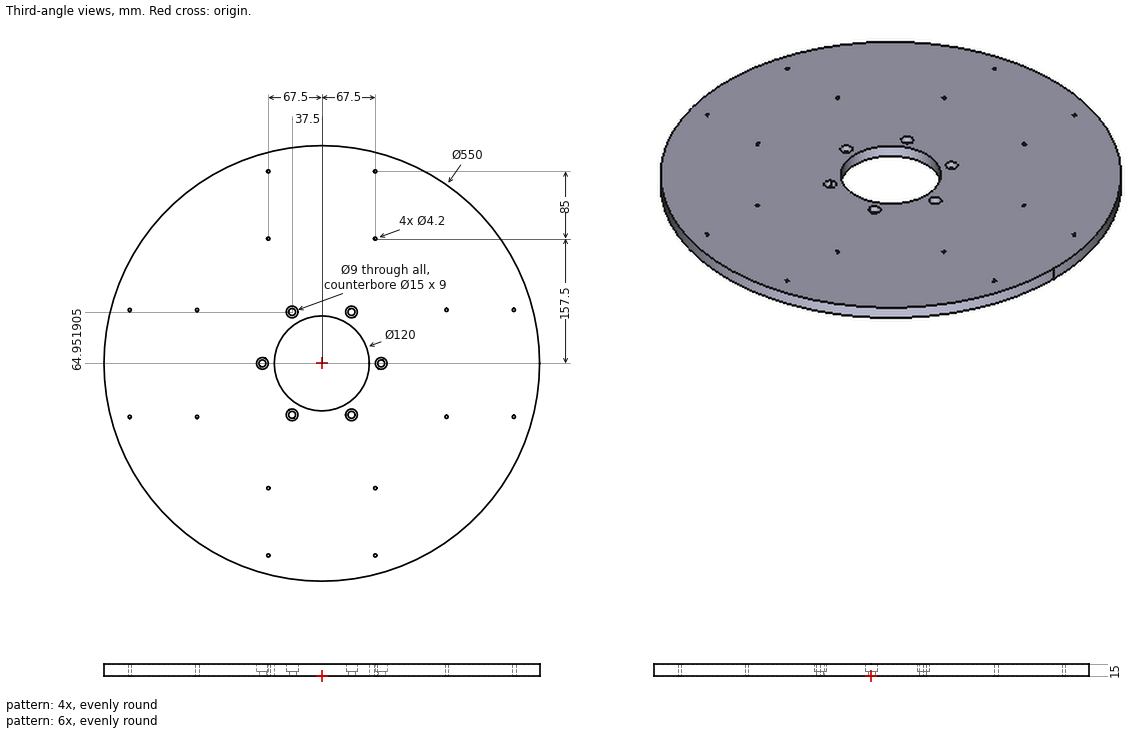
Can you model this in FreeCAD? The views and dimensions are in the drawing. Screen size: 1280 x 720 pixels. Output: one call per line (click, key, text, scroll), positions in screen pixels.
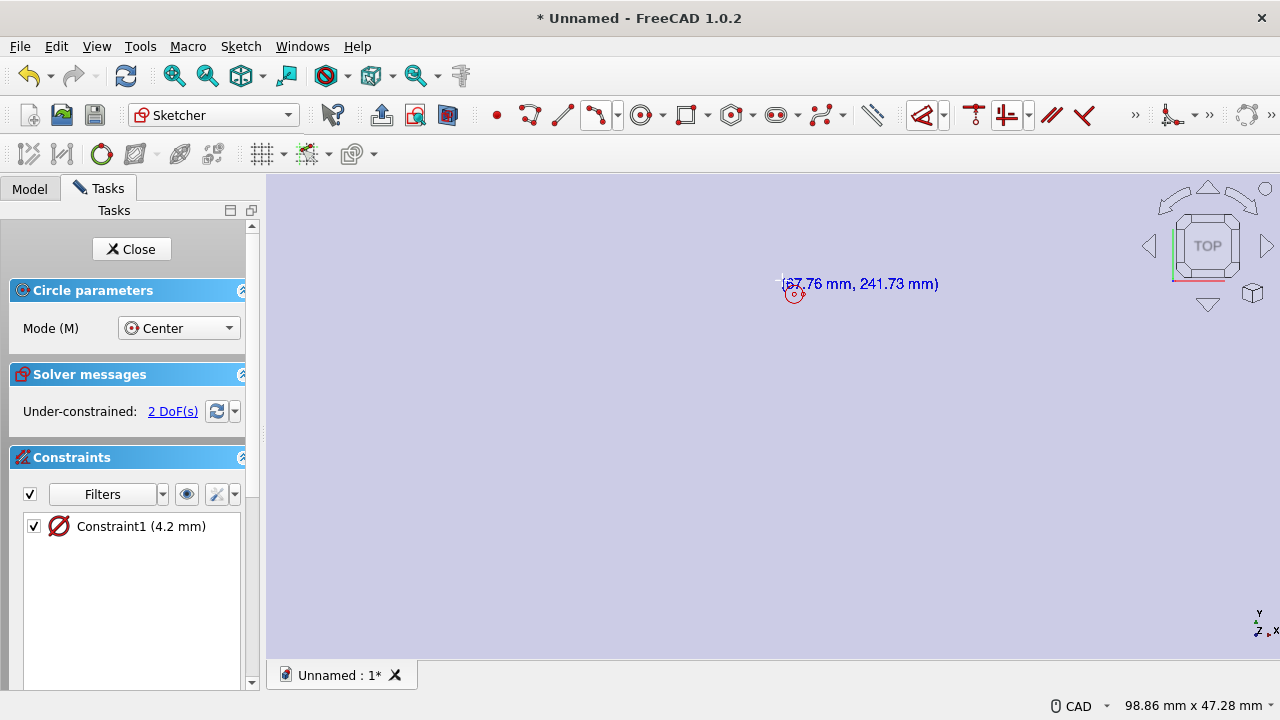
scroll(782, 280, down, 12)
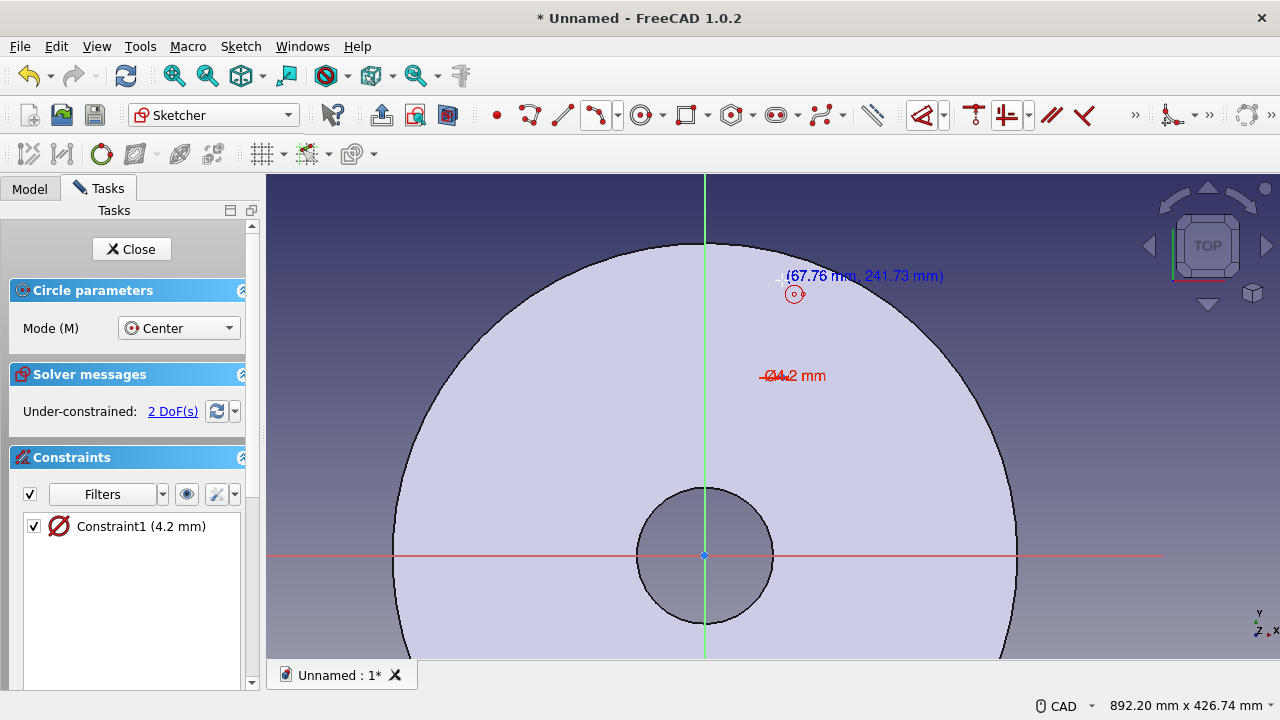
click(782, 280)
move(783, 278)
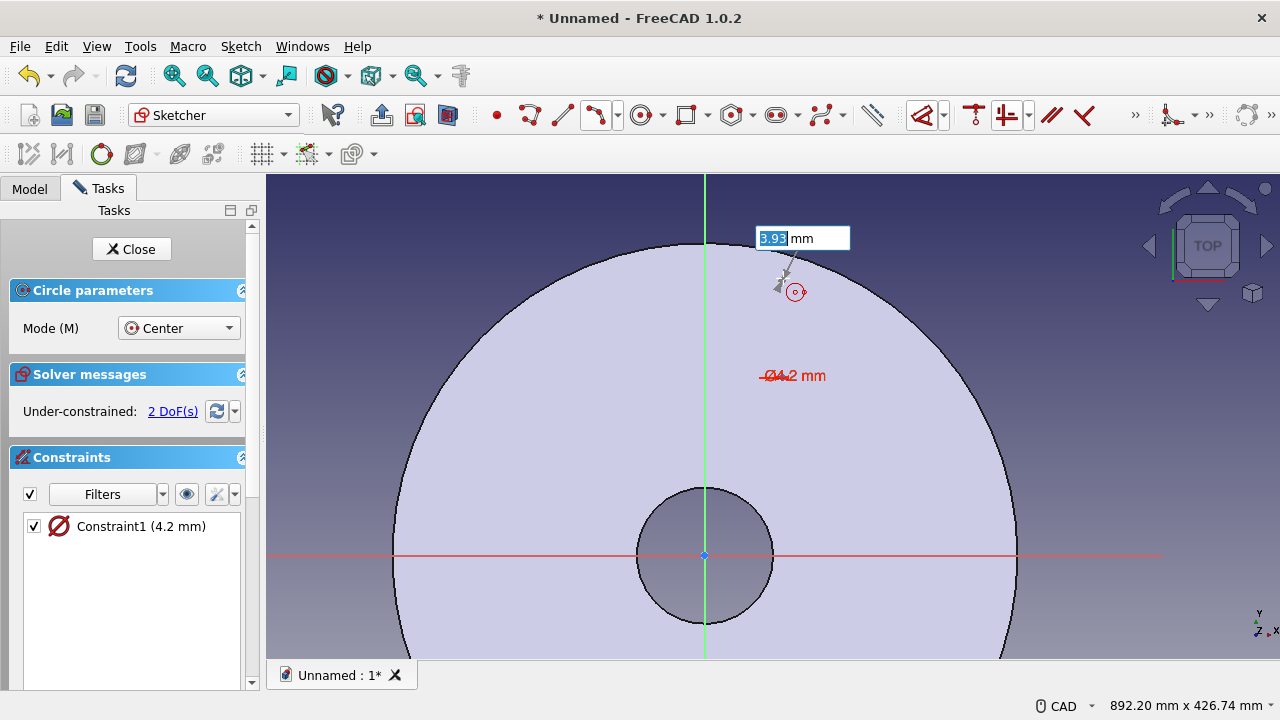
text(4.2)
key(Return)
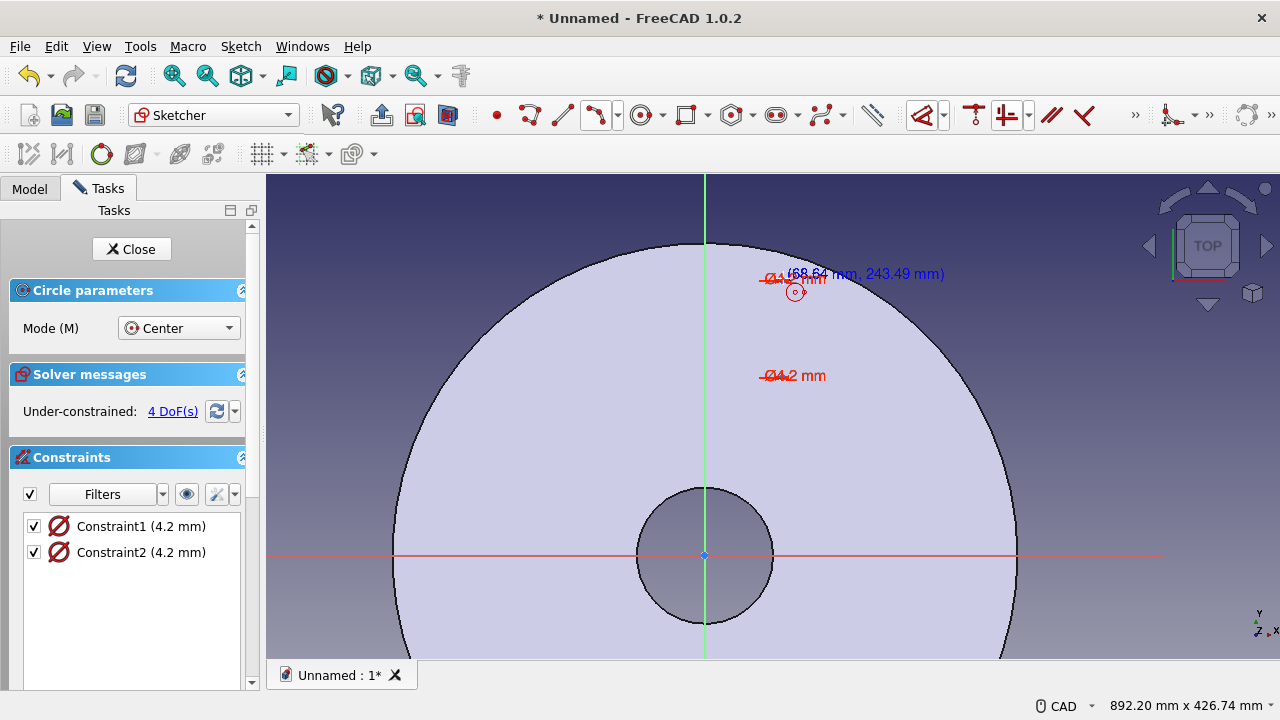
scroll(628, 377, up, 12)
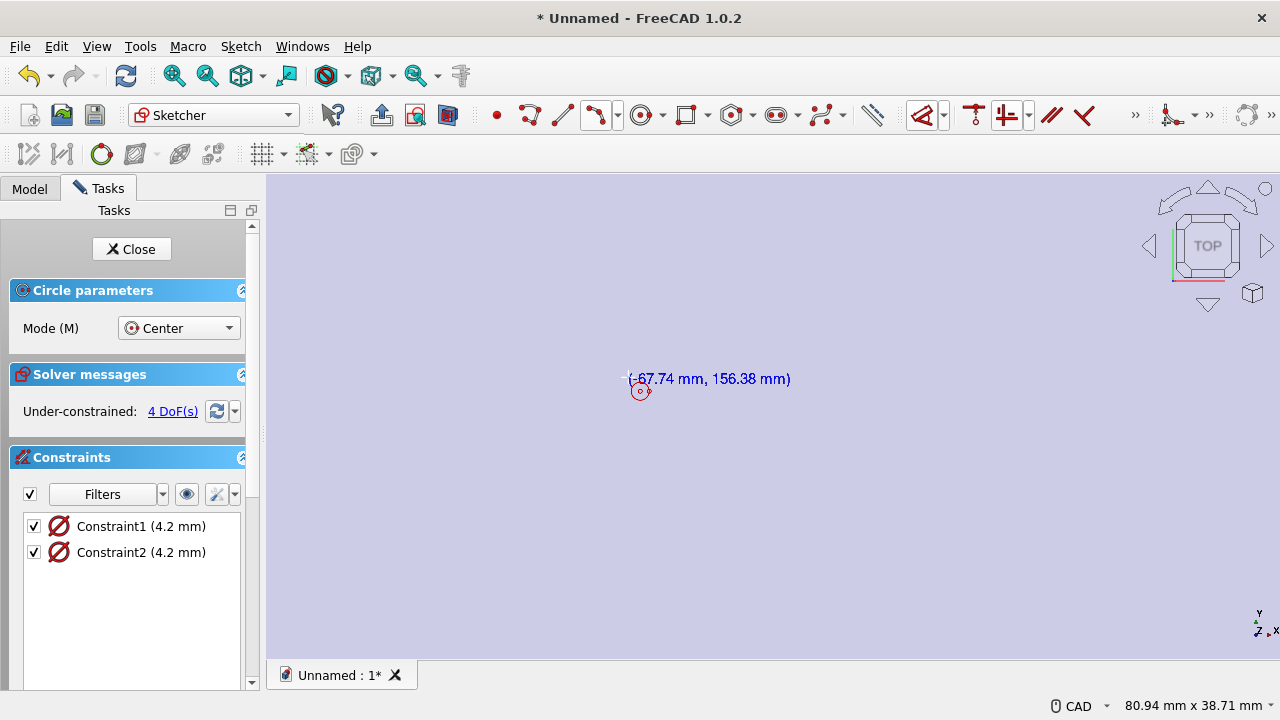
scroll(628, 377, down, 12)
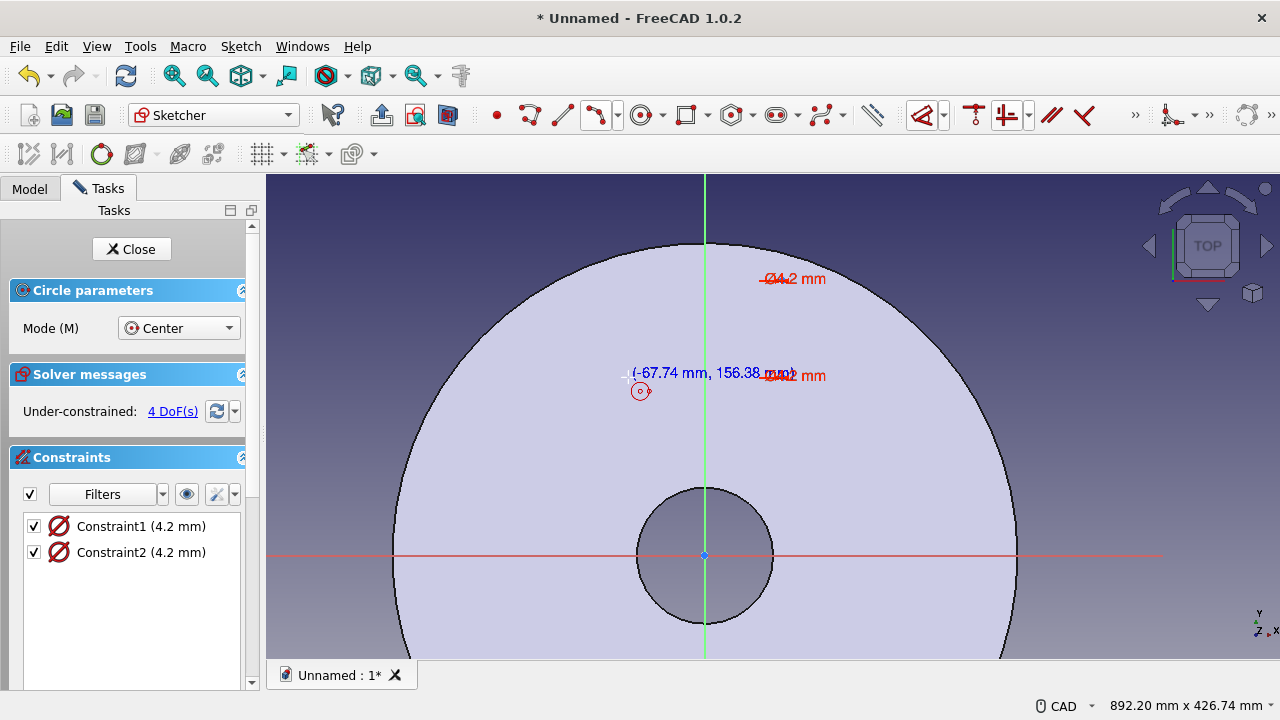
click(628, 377)
move(630, 375)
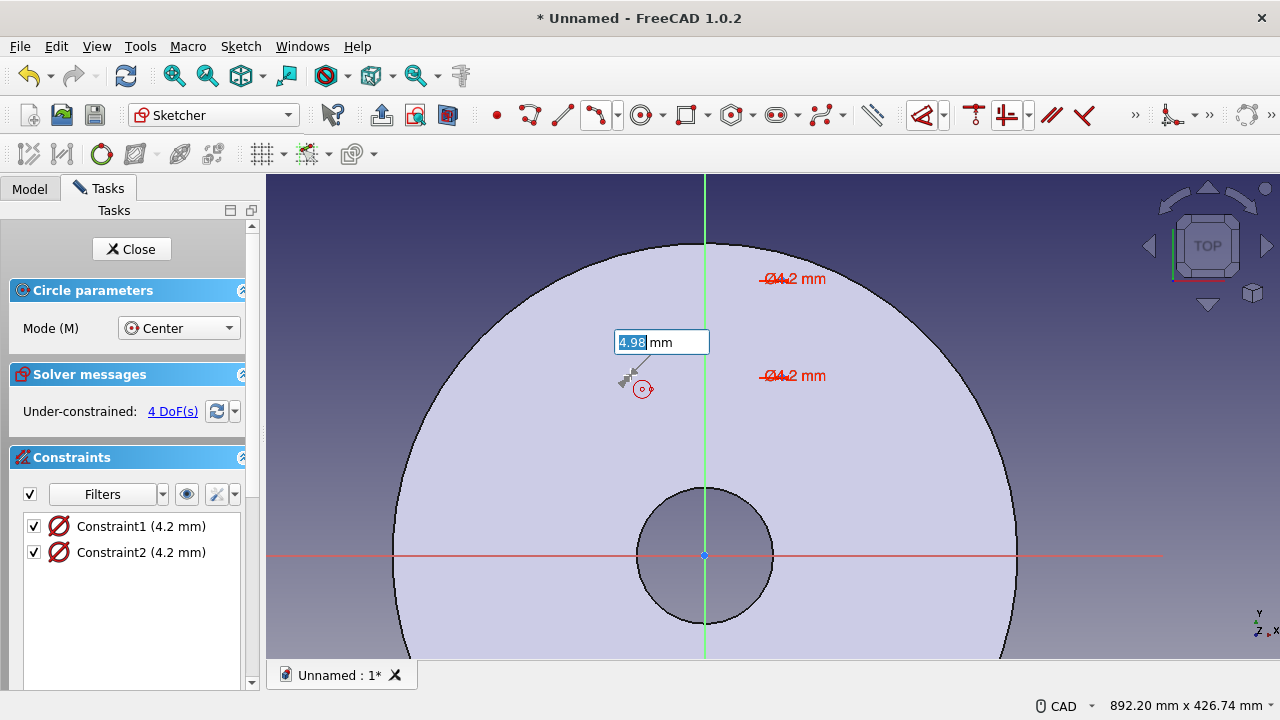
text(4.2)
key(Return)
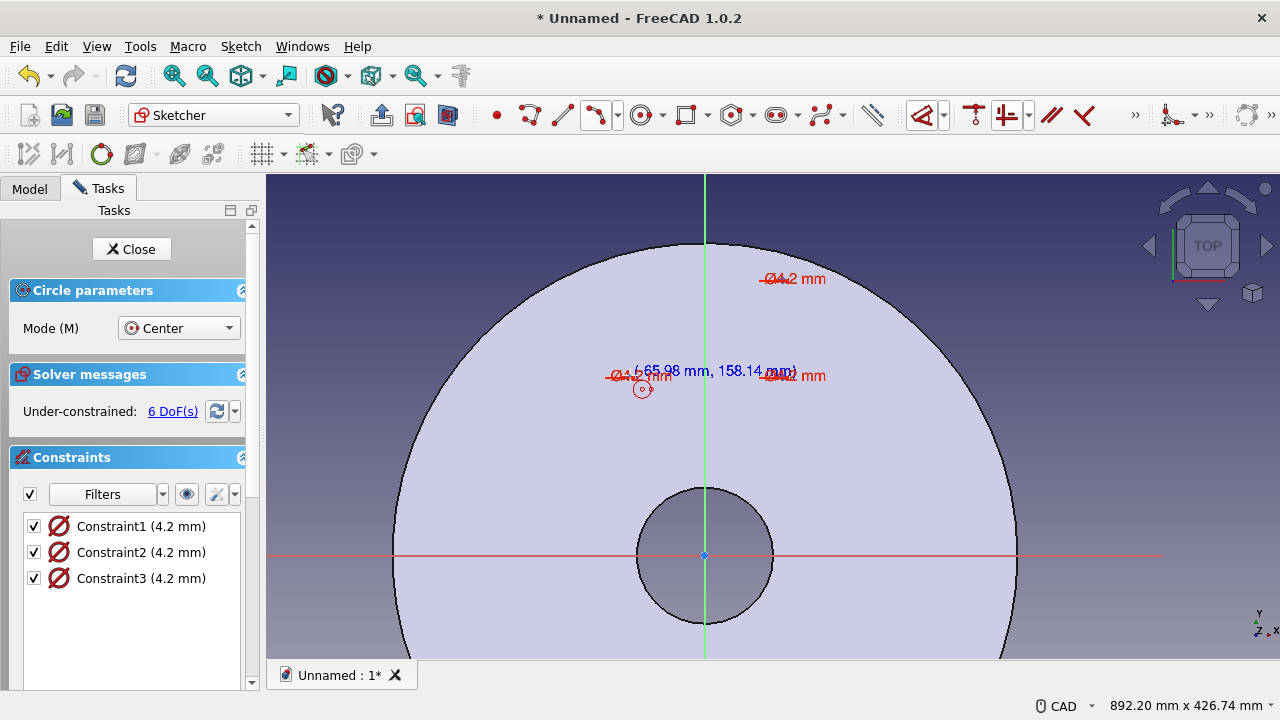
scroll(628, 280, up, 12)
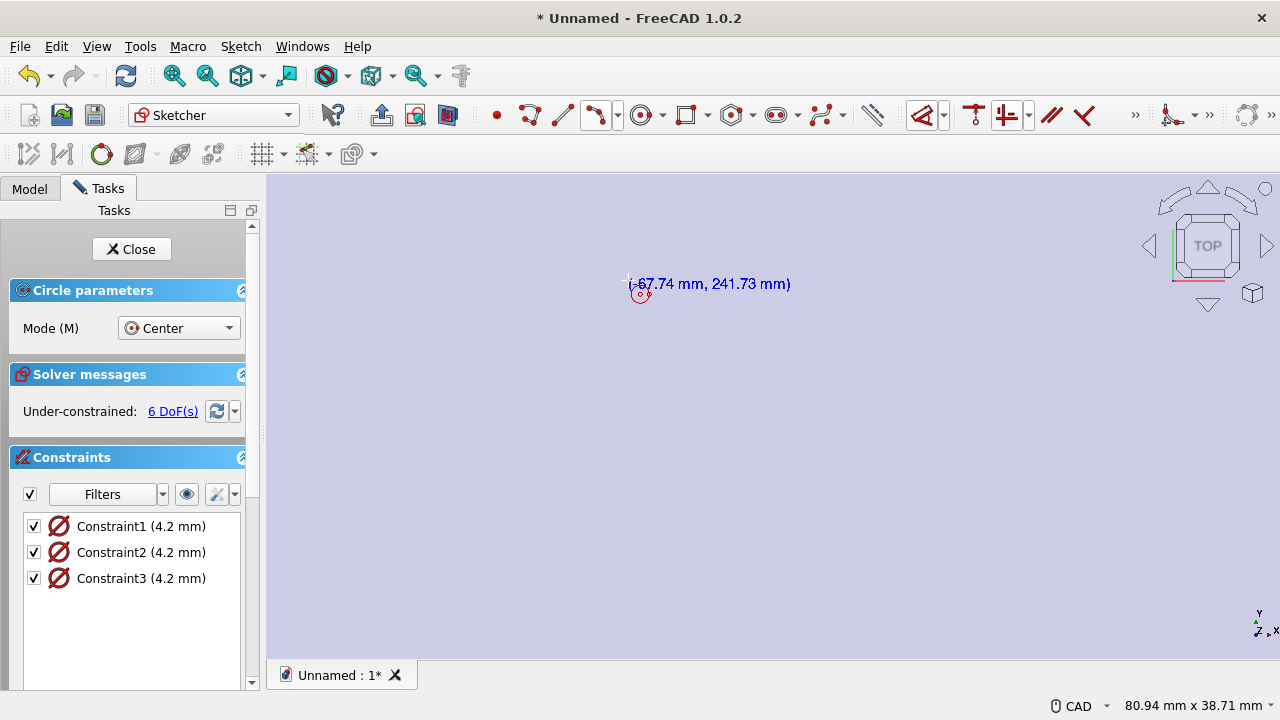
scroll(628, 280, down, 12)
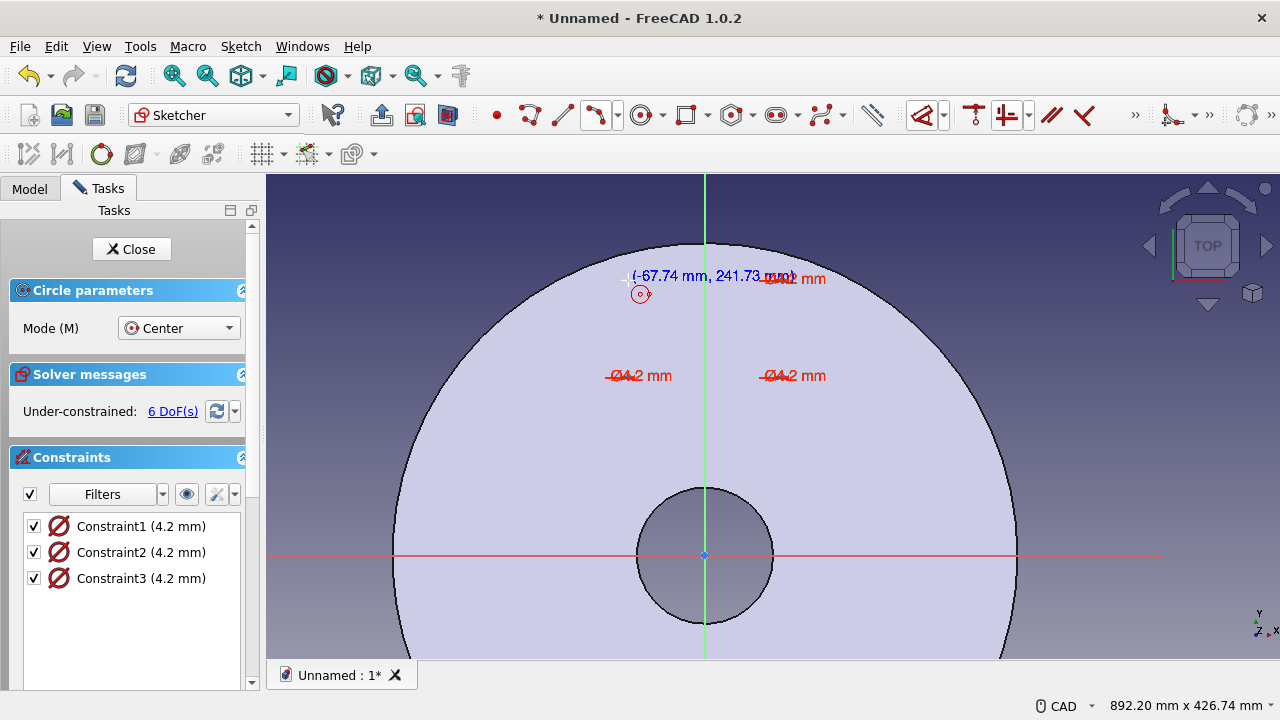
click(628, 280)
move(630, 278)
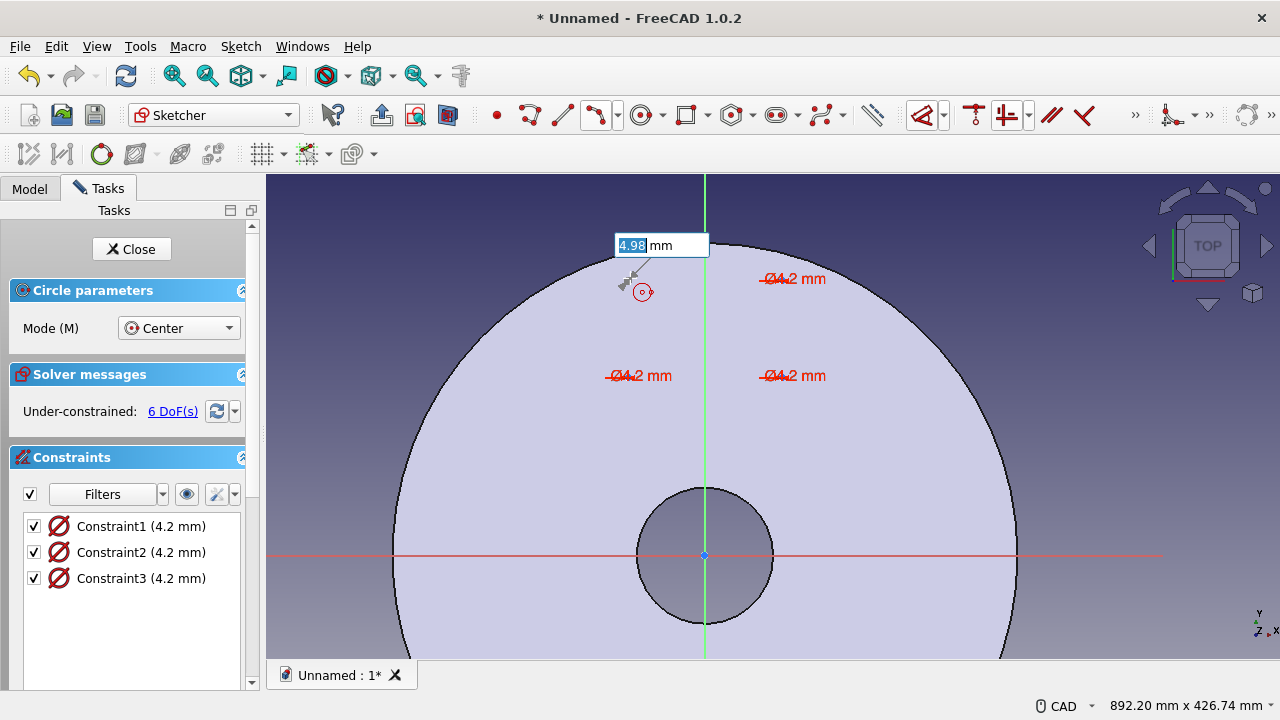
text(4.2)
key(Return)
key(Escape)